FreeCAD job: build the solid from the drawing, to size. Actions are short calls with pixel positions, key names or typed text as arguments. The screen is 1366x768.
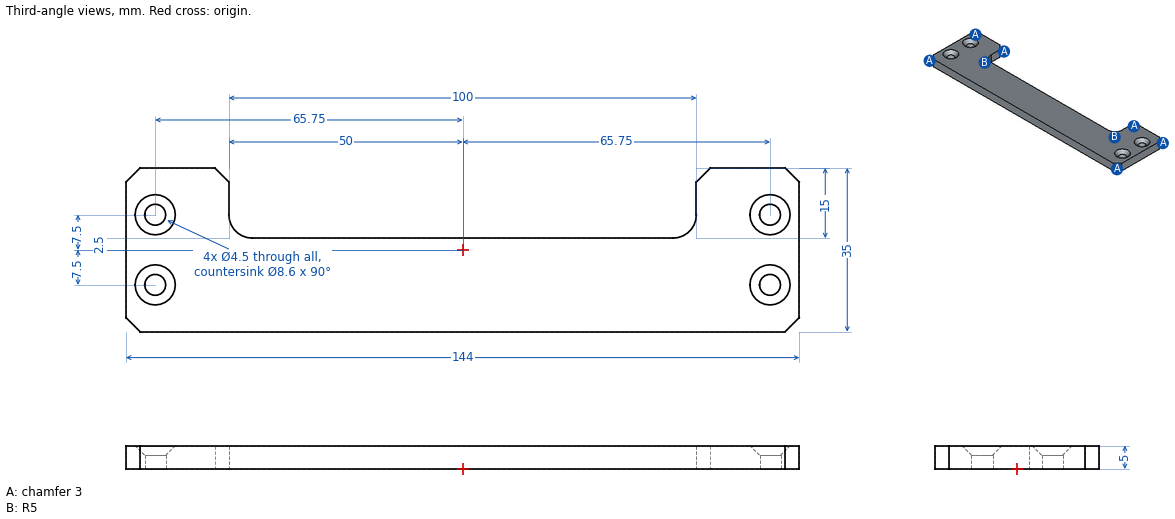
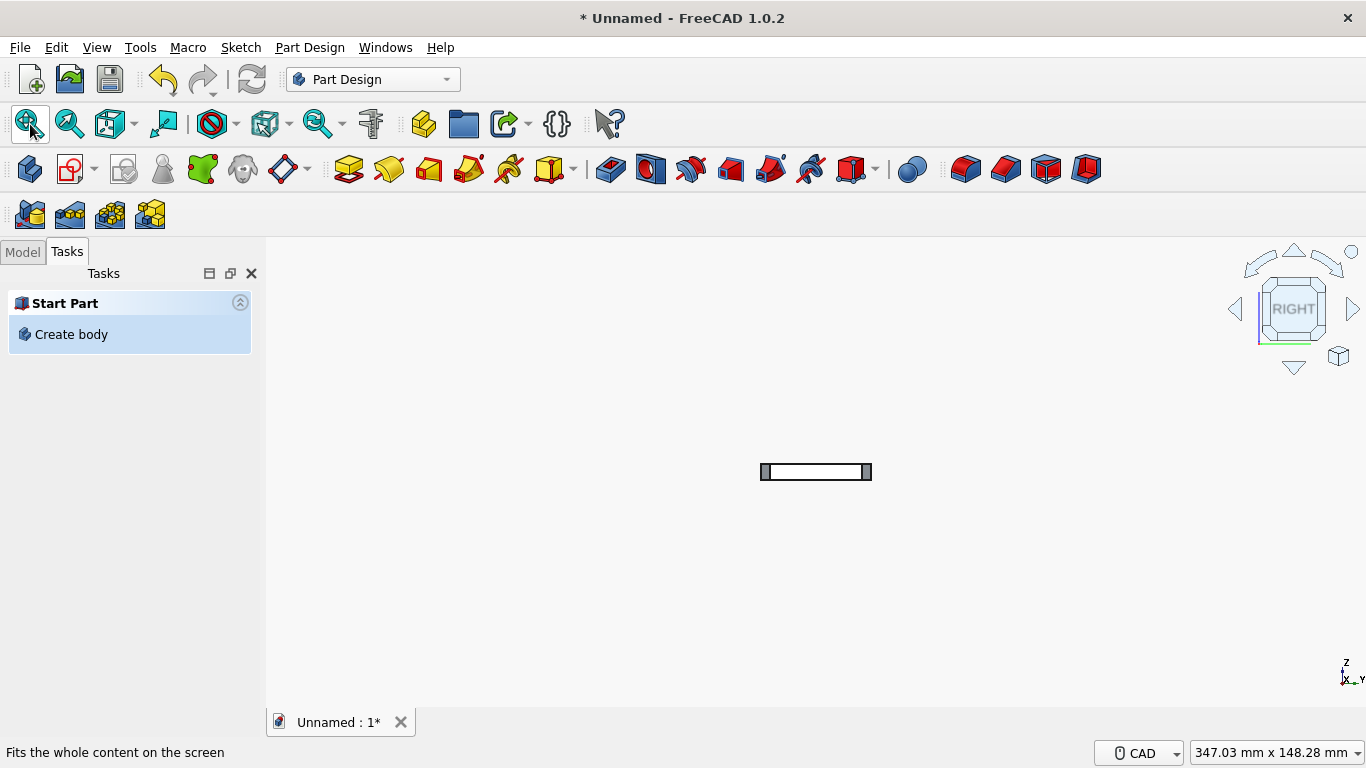
key(v)
key(f)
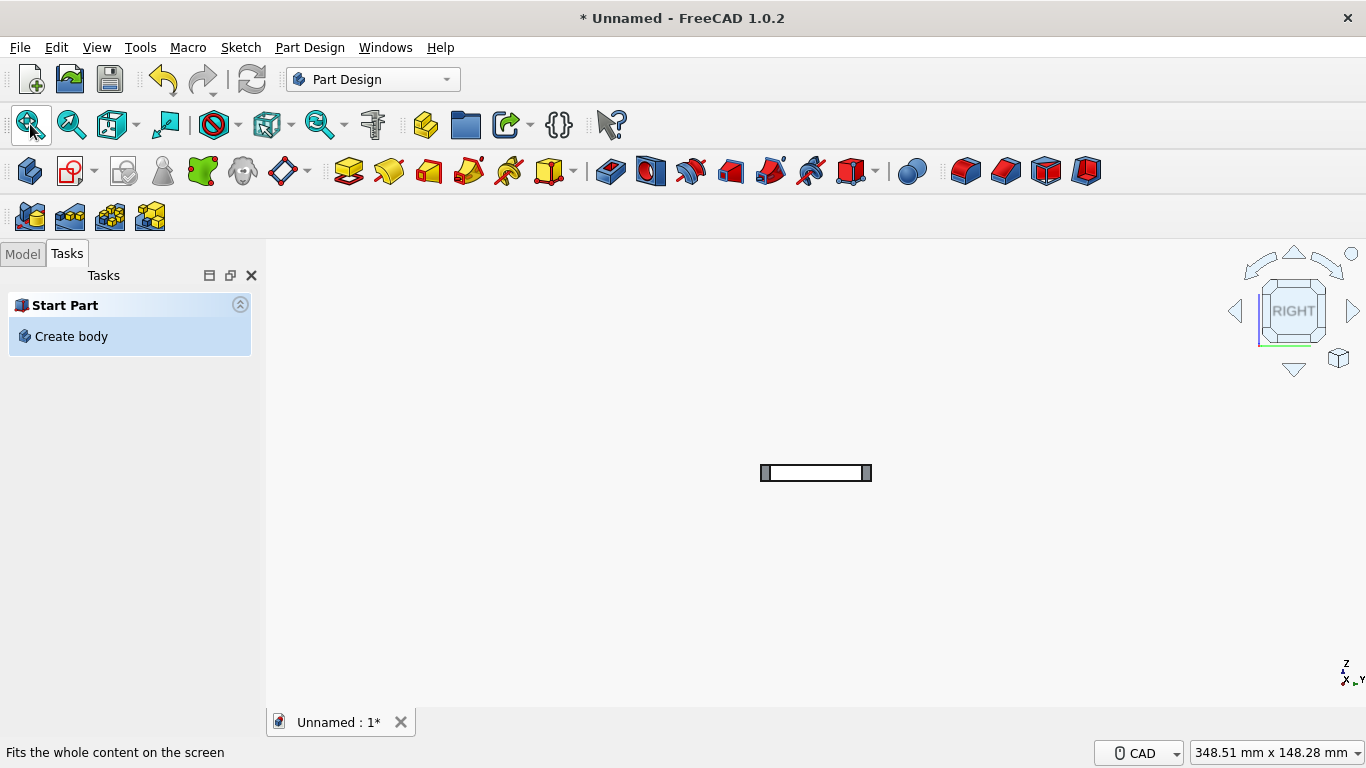
scroll(824, 472, up, 5)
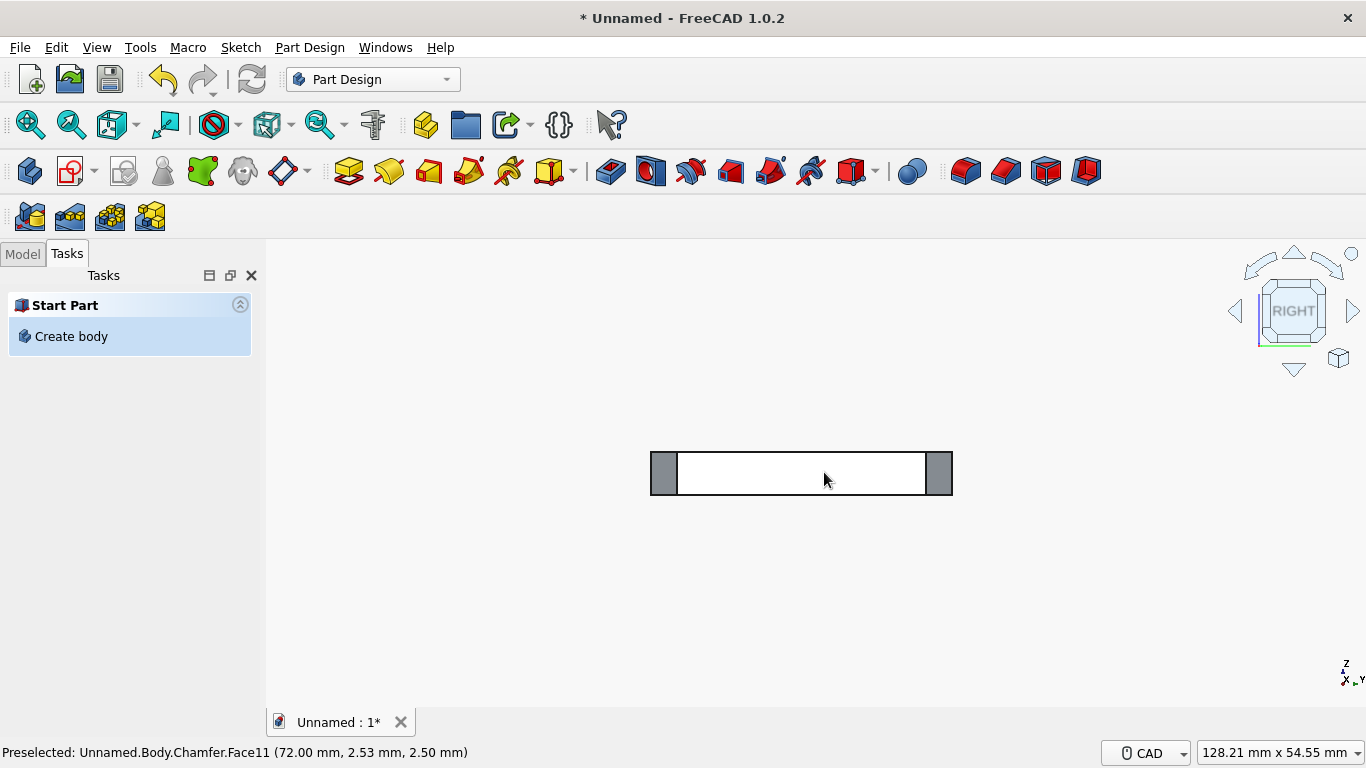
click(32, 126)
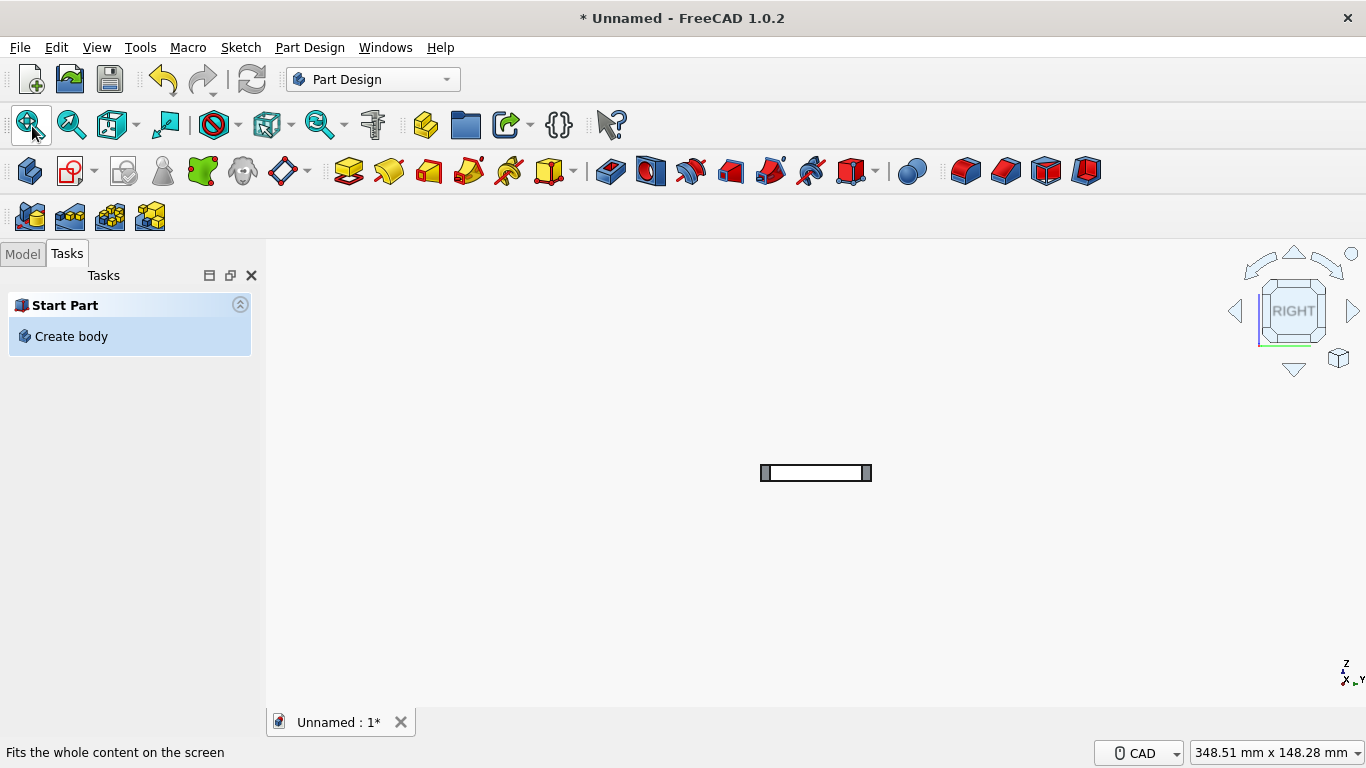
key(5)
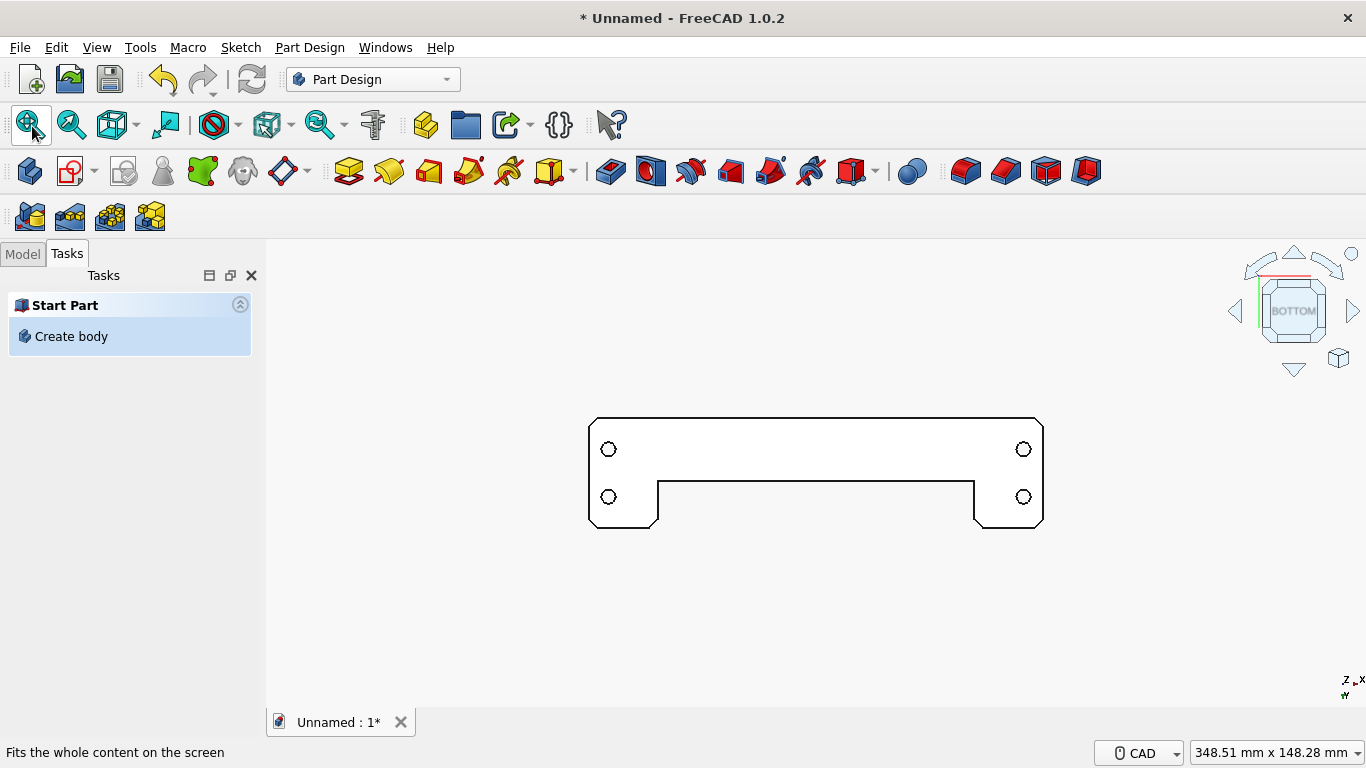
click(32, 126)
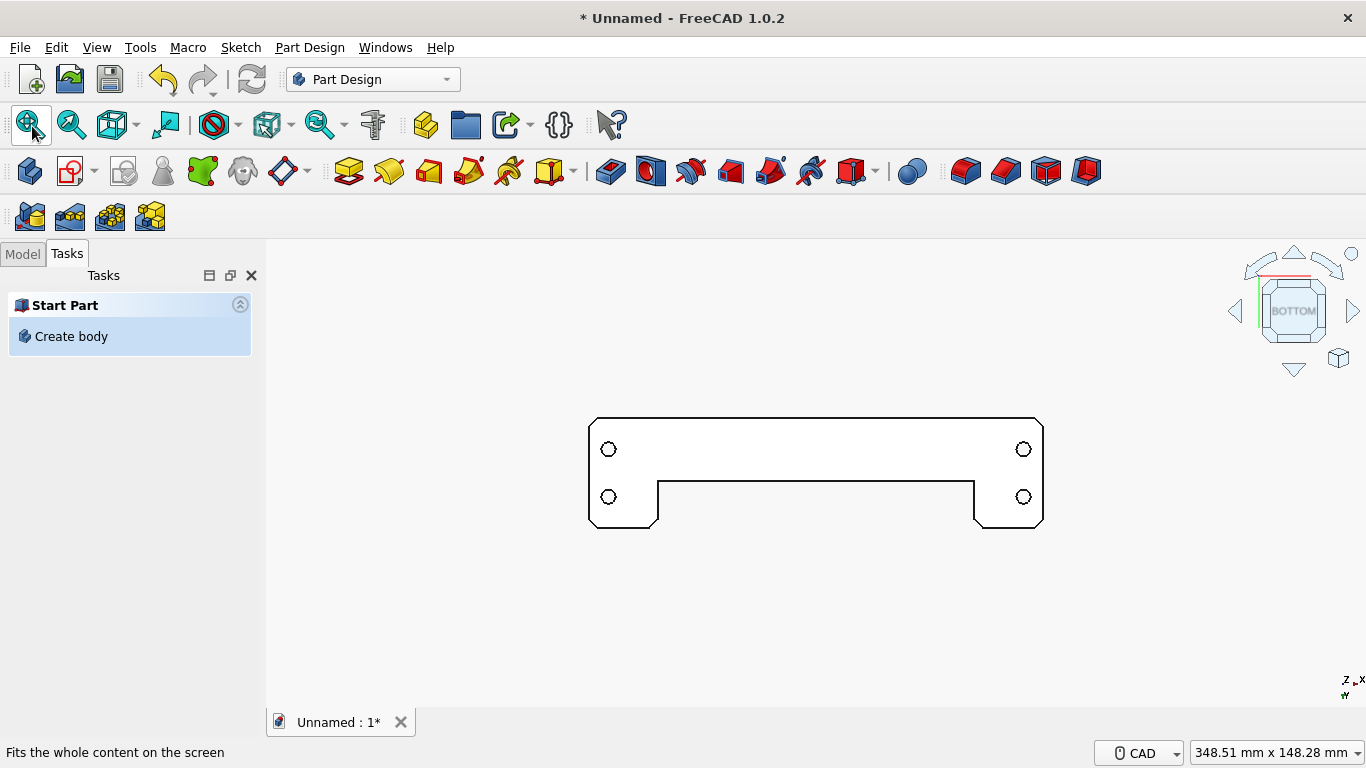
scroll(658, 480, up, 5)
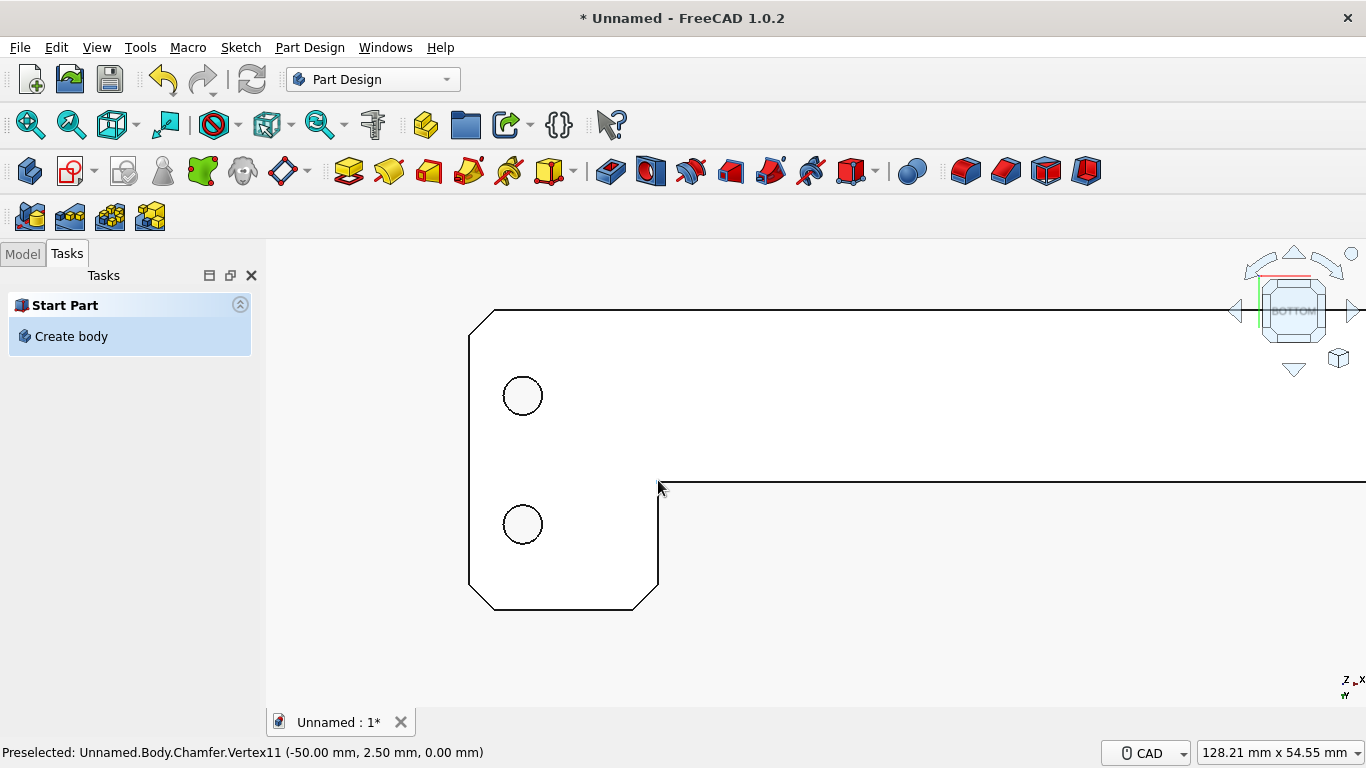
key(v)
key(f)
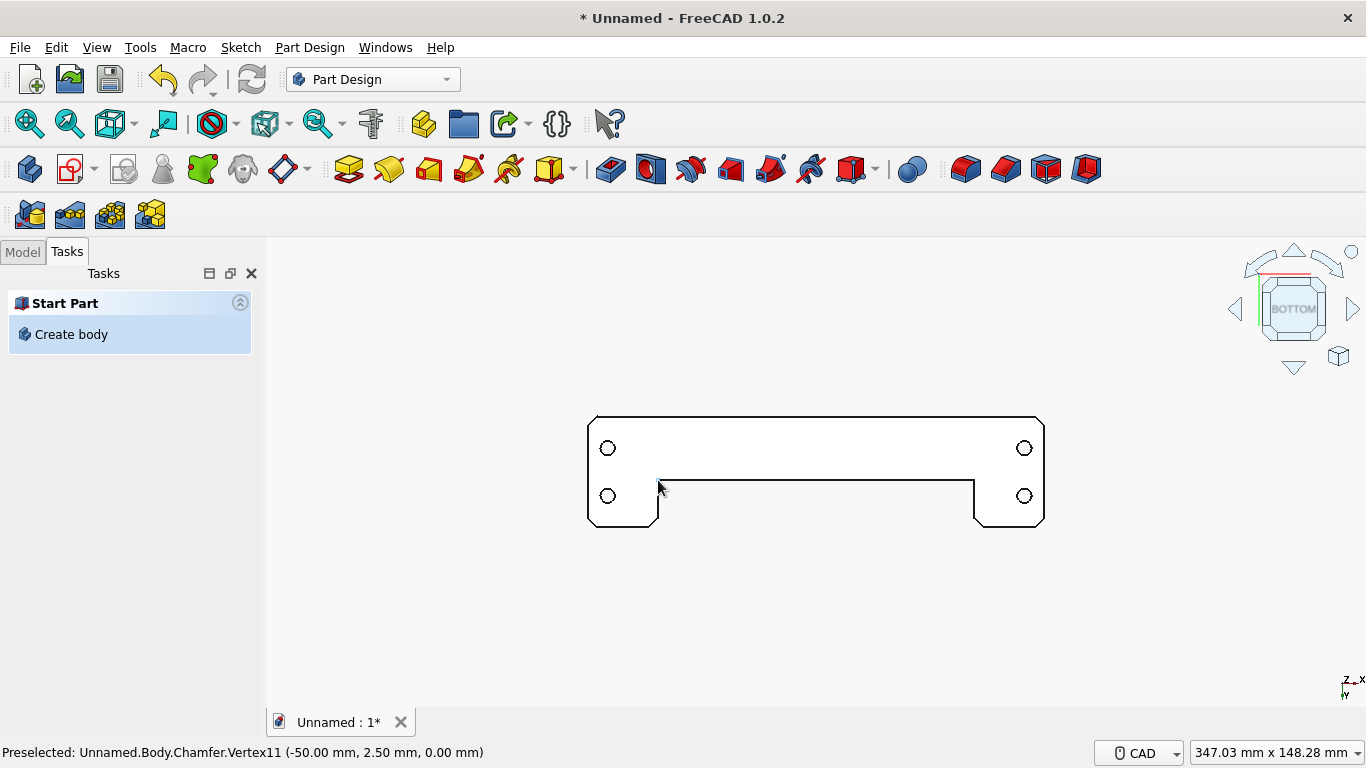
key(4)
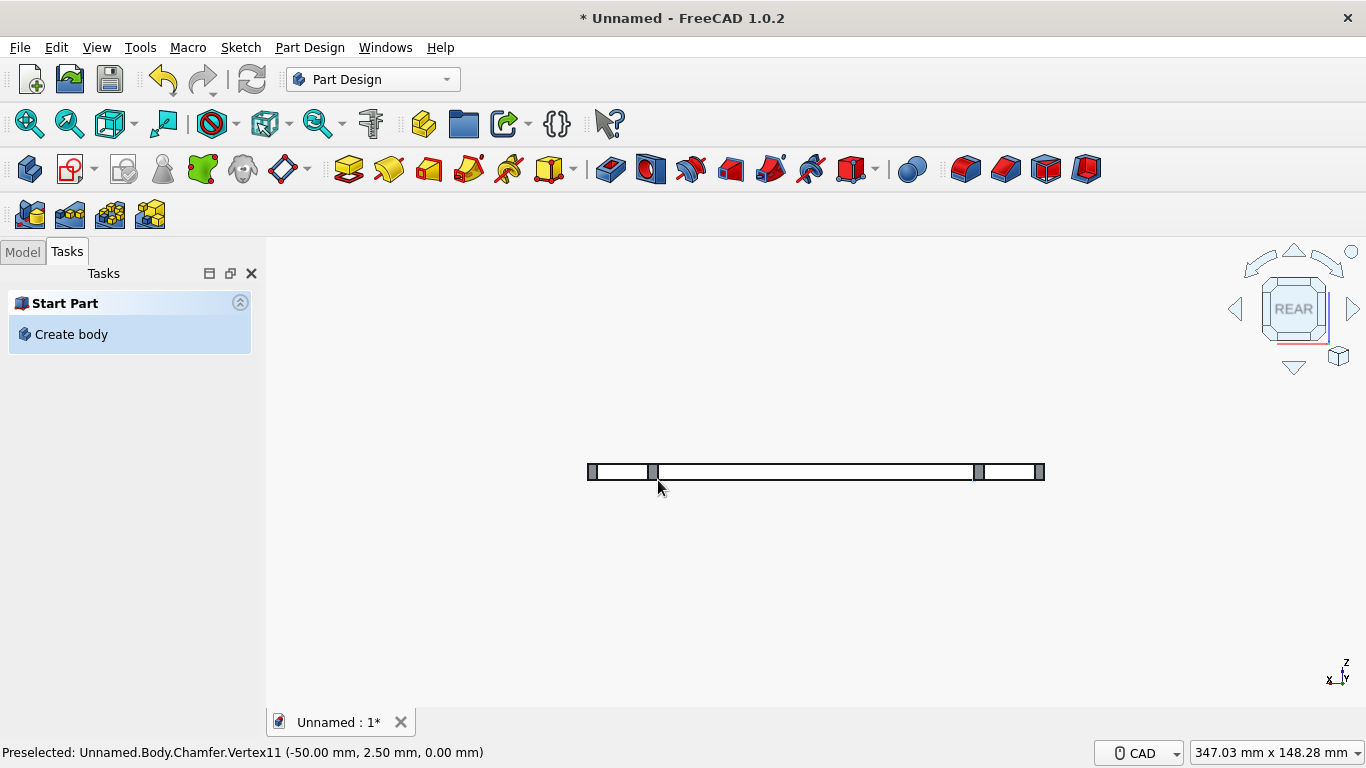
key(v)
key(f)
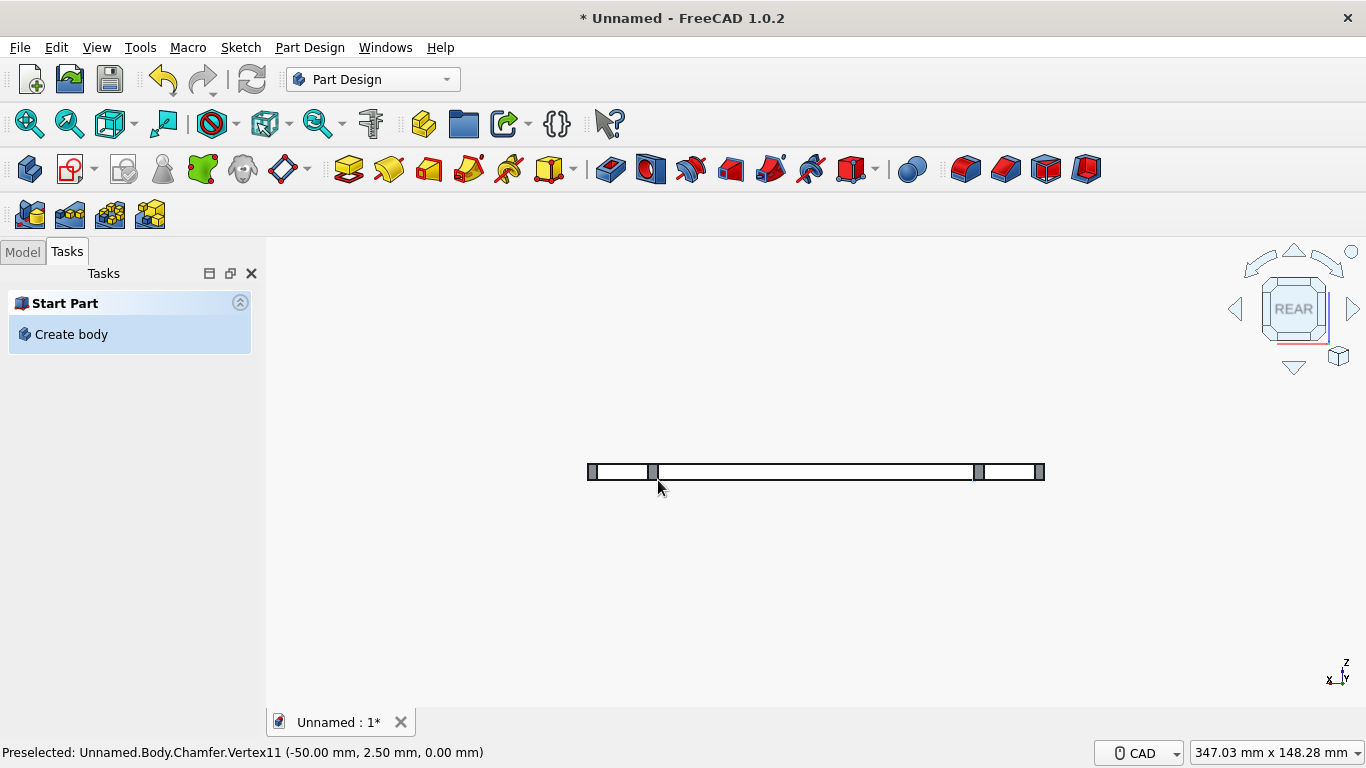
scroll(974, 471, up, 5)